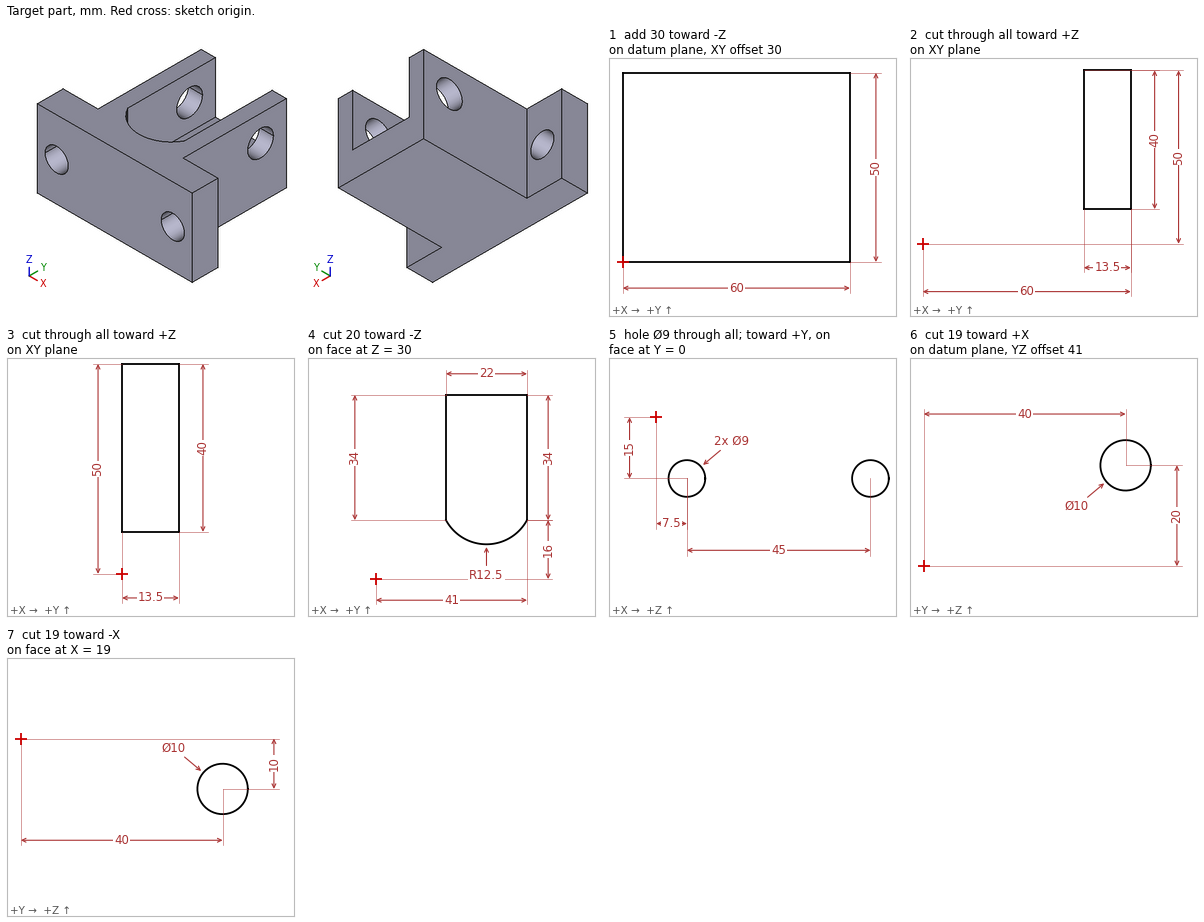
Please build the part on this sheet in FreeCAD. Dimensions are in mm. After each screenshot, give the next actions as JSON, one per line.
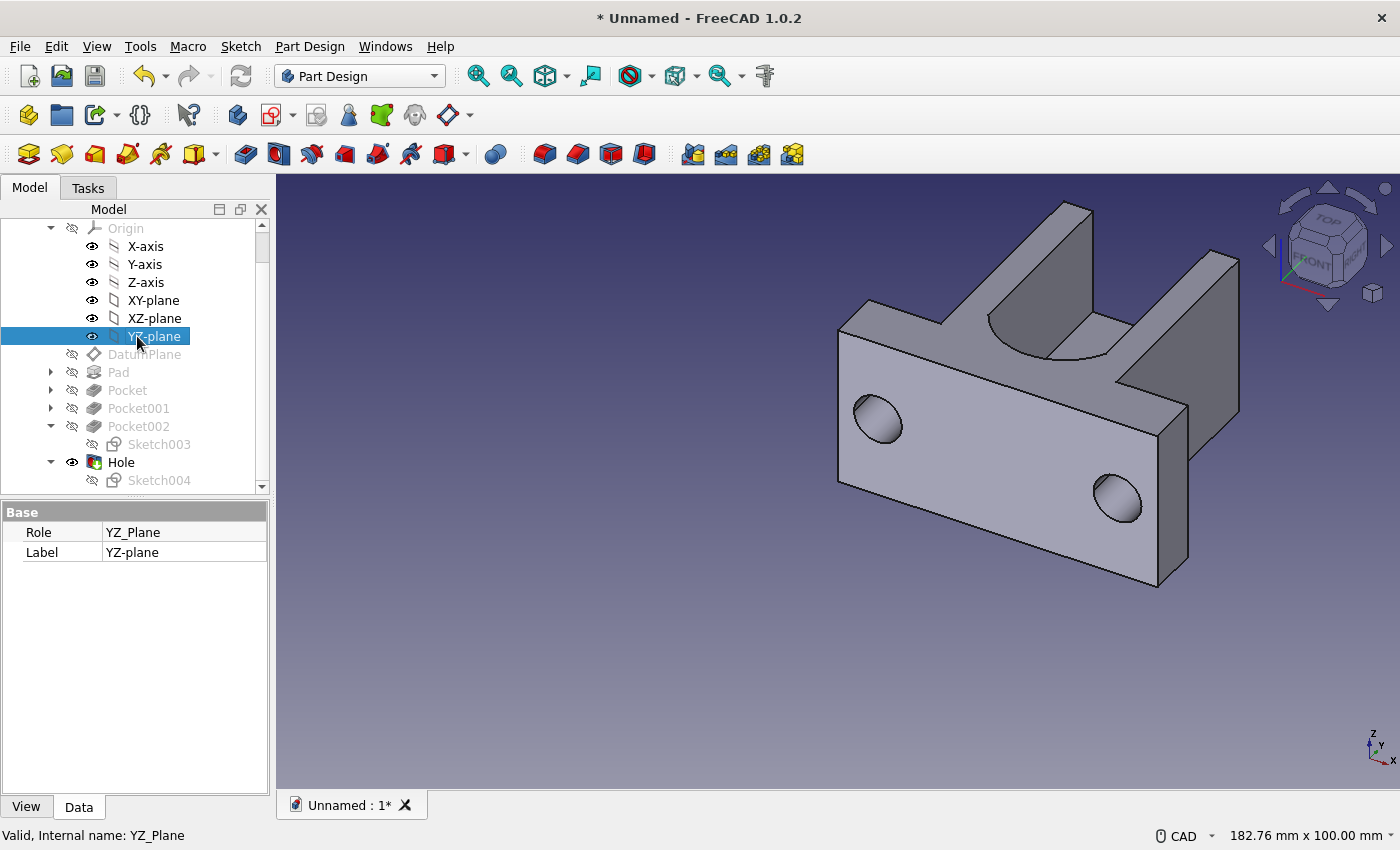
{"action": "left_click", "coordinate": [448, 116]}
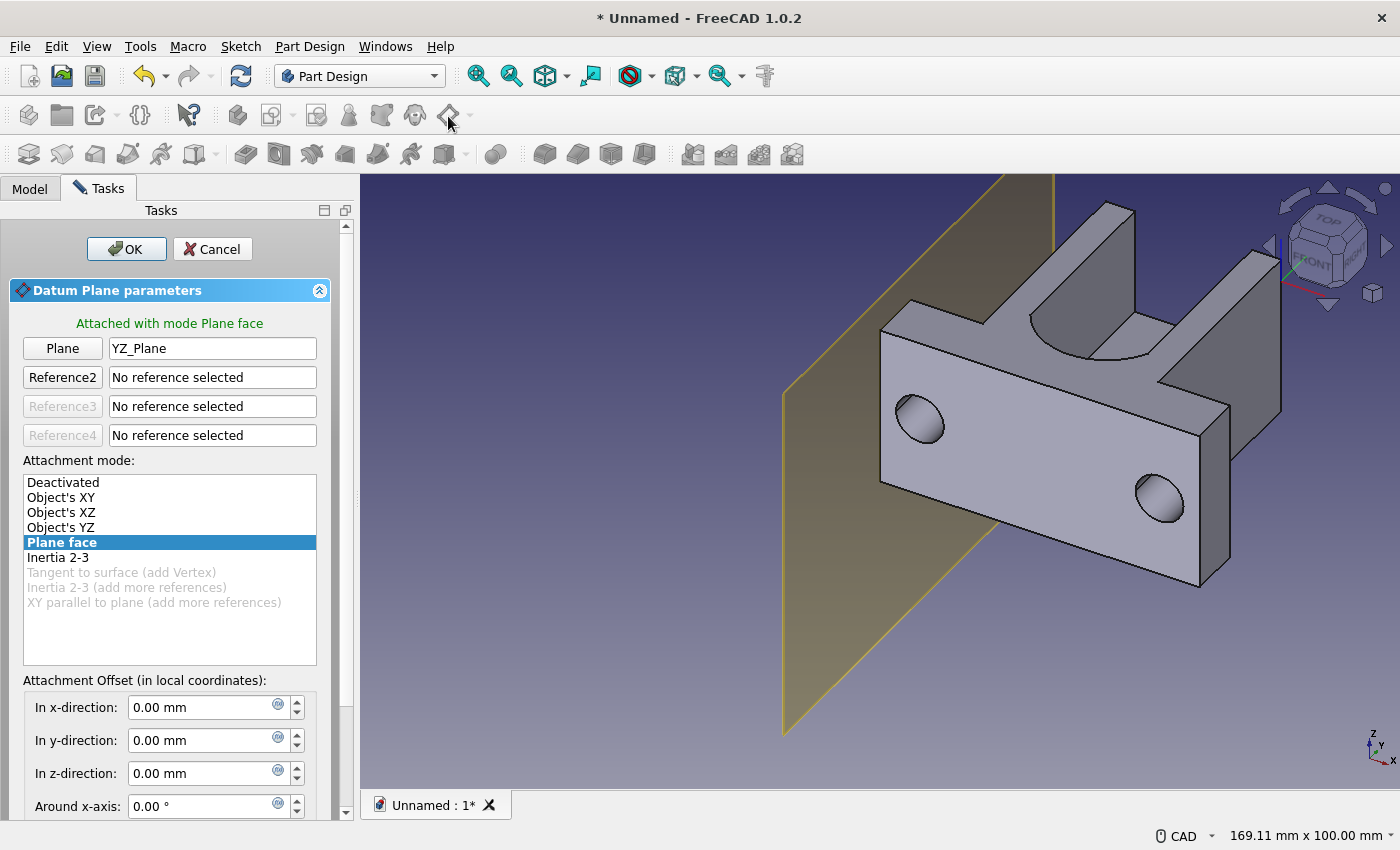
{"action": "triple_click", "coordinate": [210, 774]}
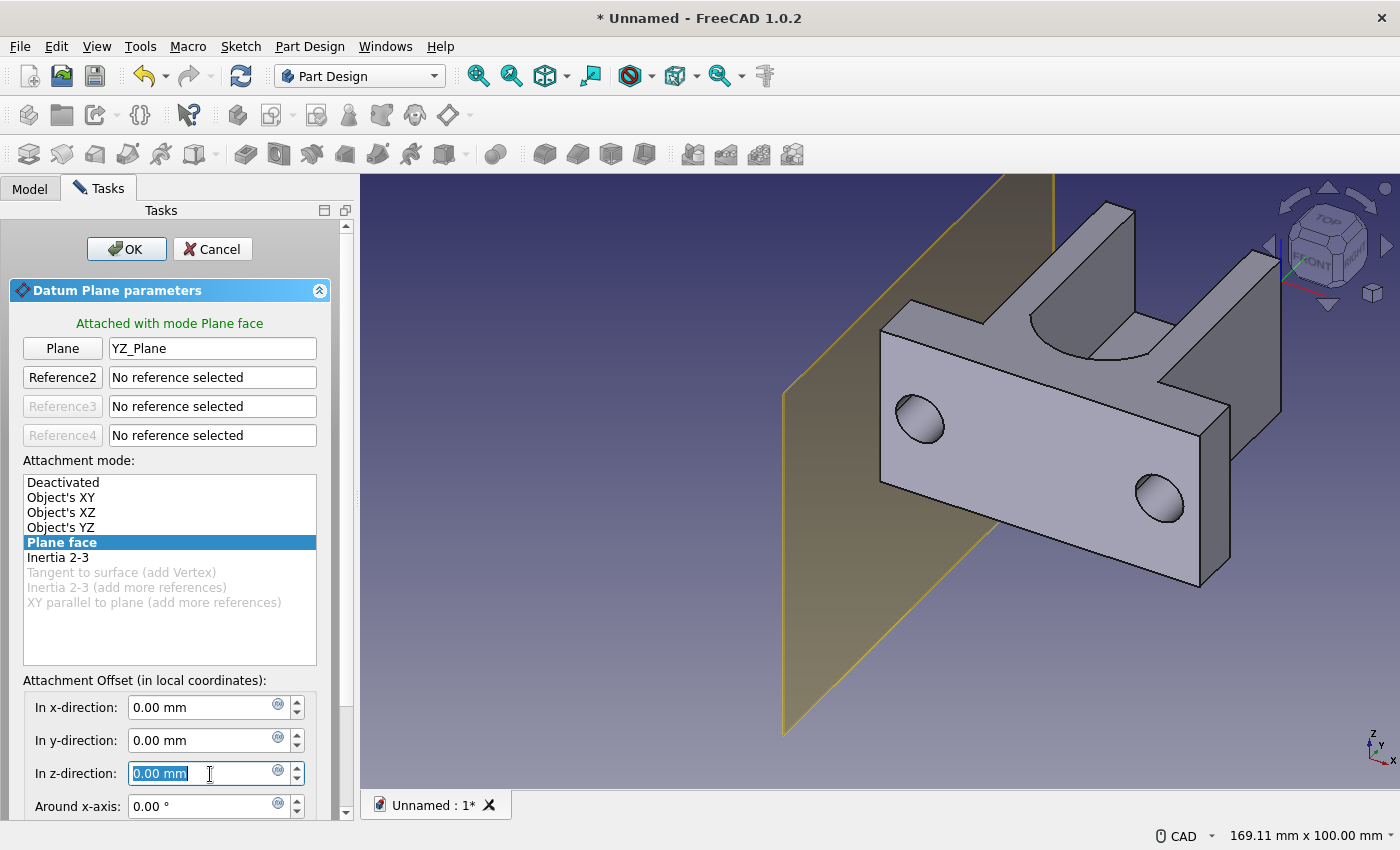
{"action": "type", "text": "41"}
{"action": "key", "text": "Tab"}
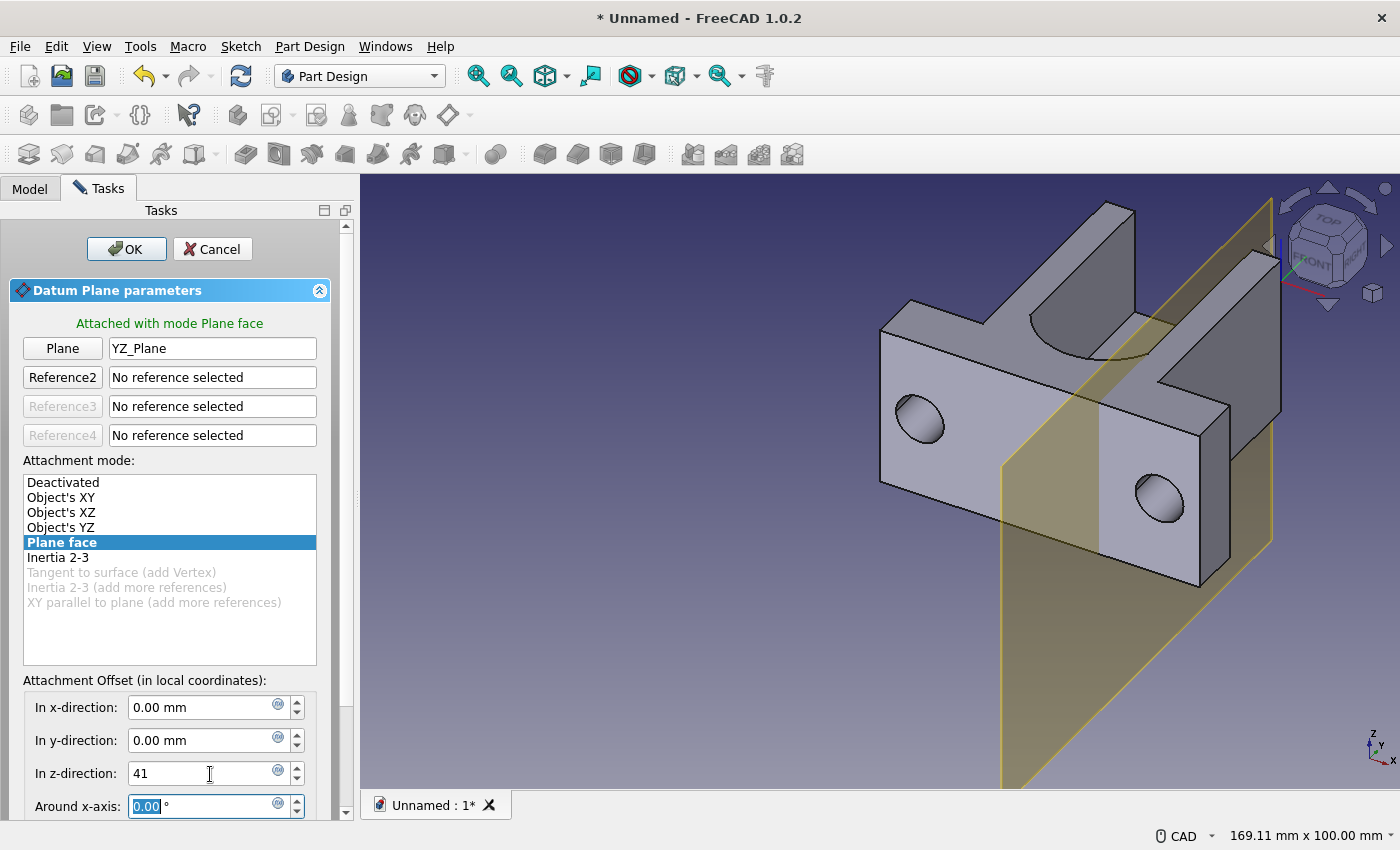
{"action": "left_click", "coordinate": [127, 249]}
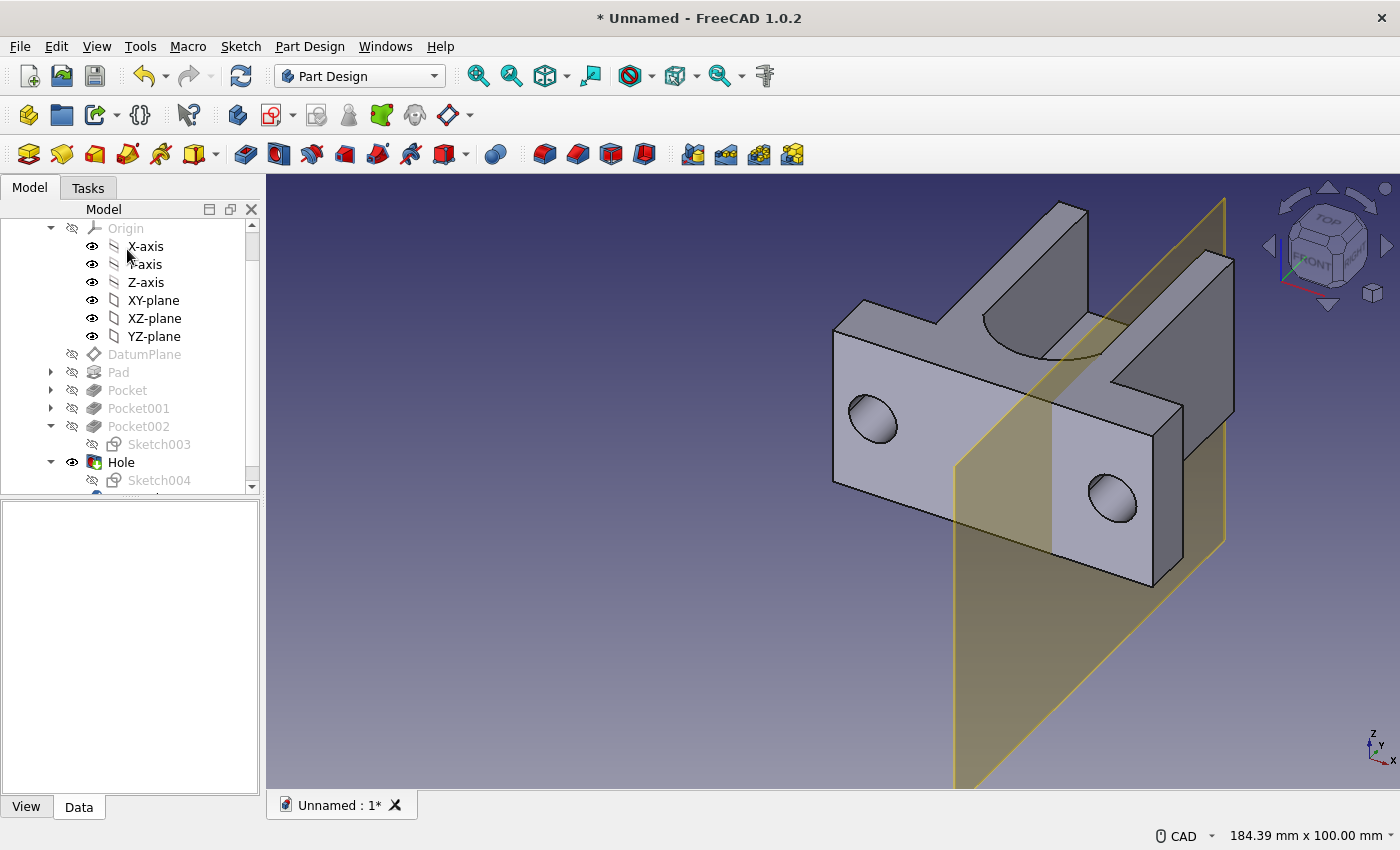
{"action": "scroll", "coordinate": [141, 350], "scroll_direction": "down", "scroll_amount": 3}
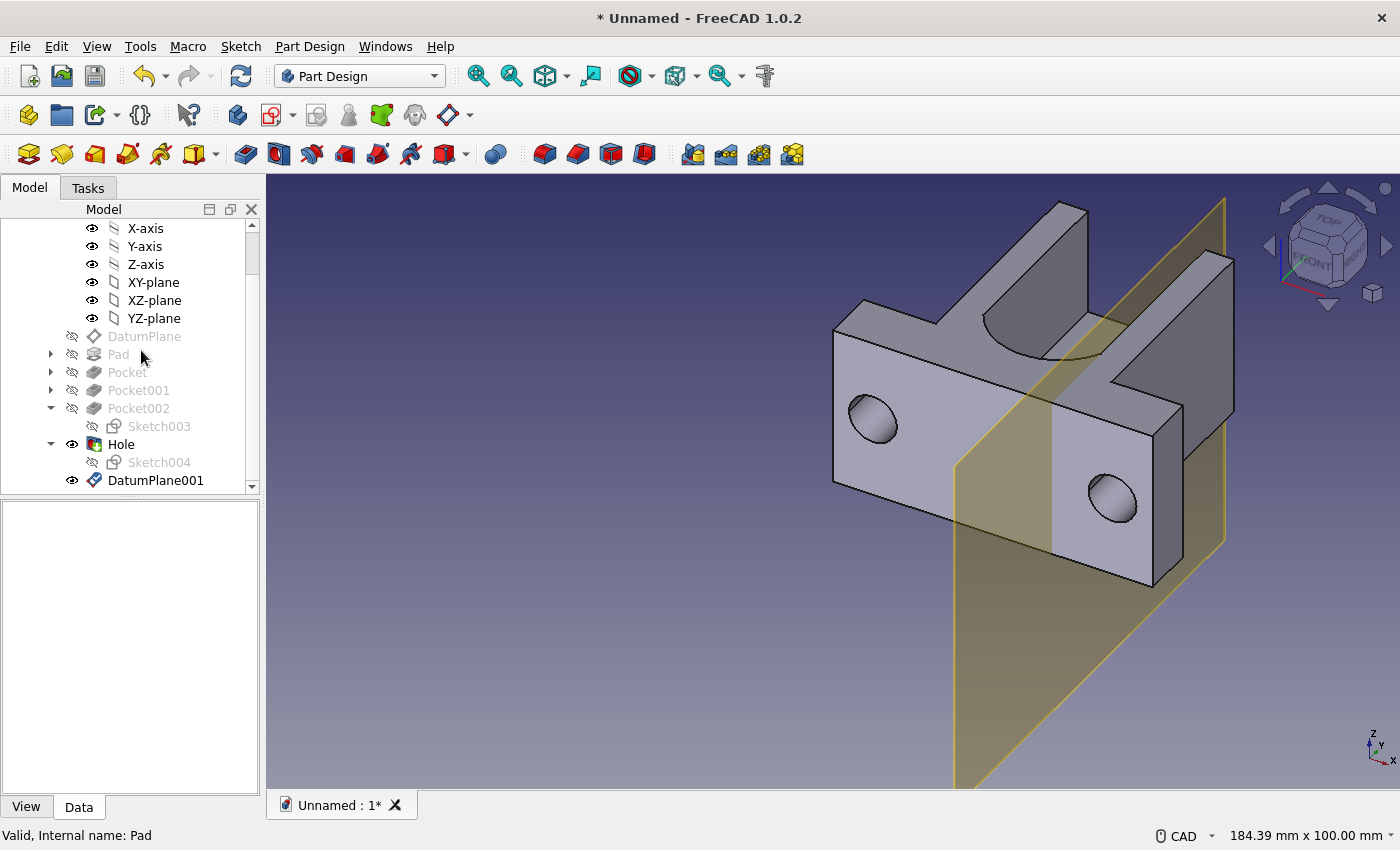
{"action": "left_click", "coordinate": [117, 480]}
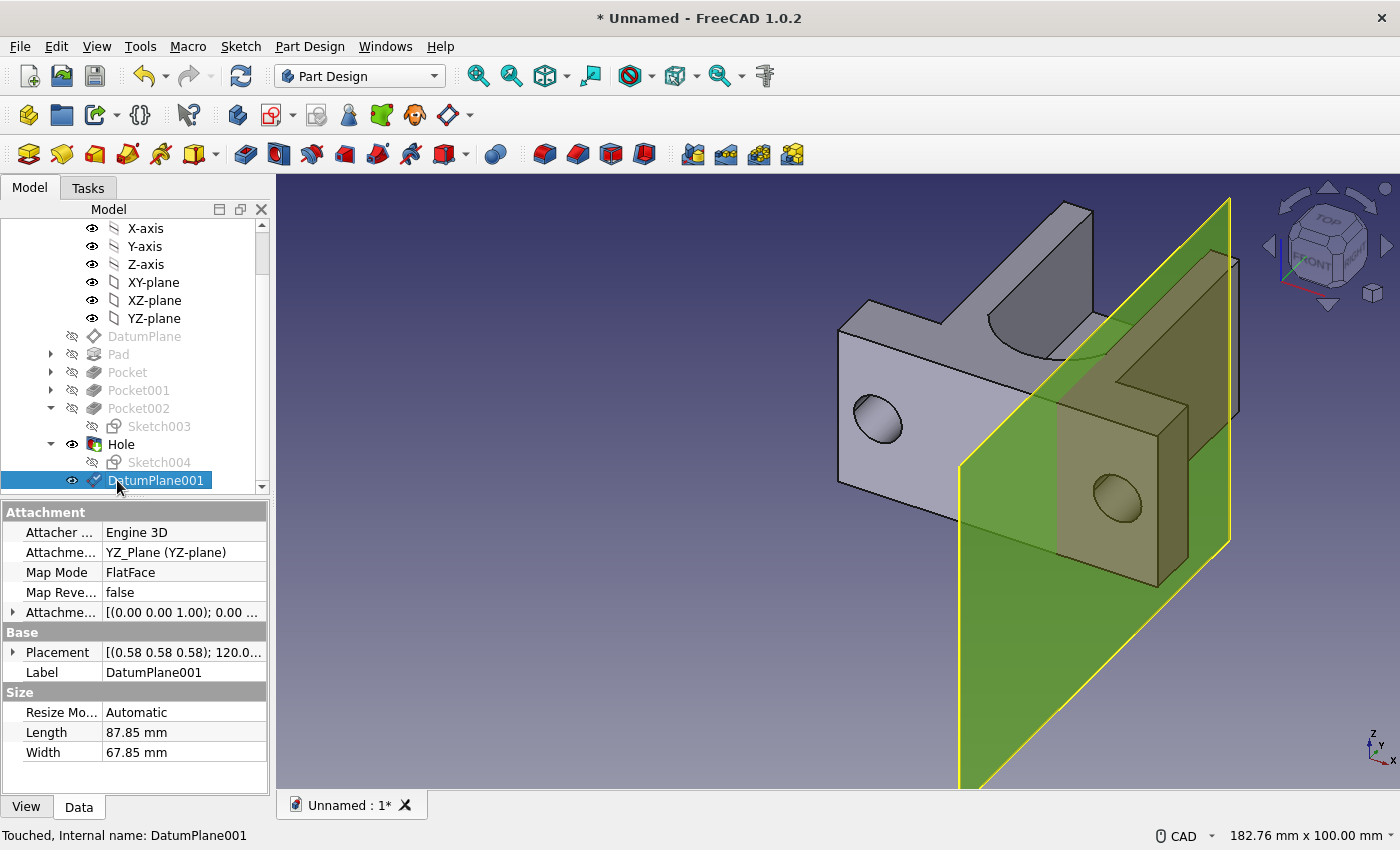
{"action": "left_click", "coordinate": [270, 116]}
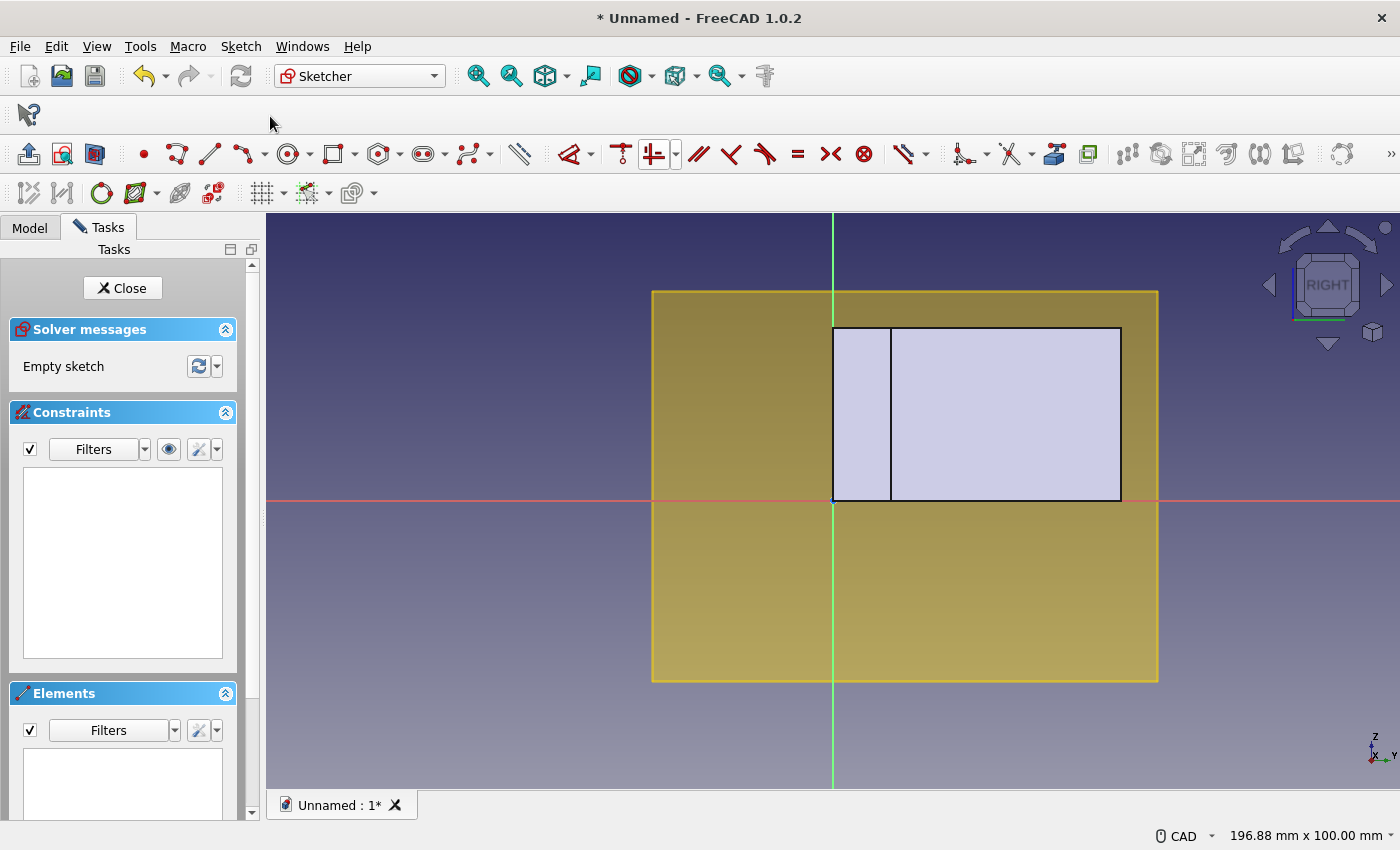
{"action": "key", "text": "q s"}